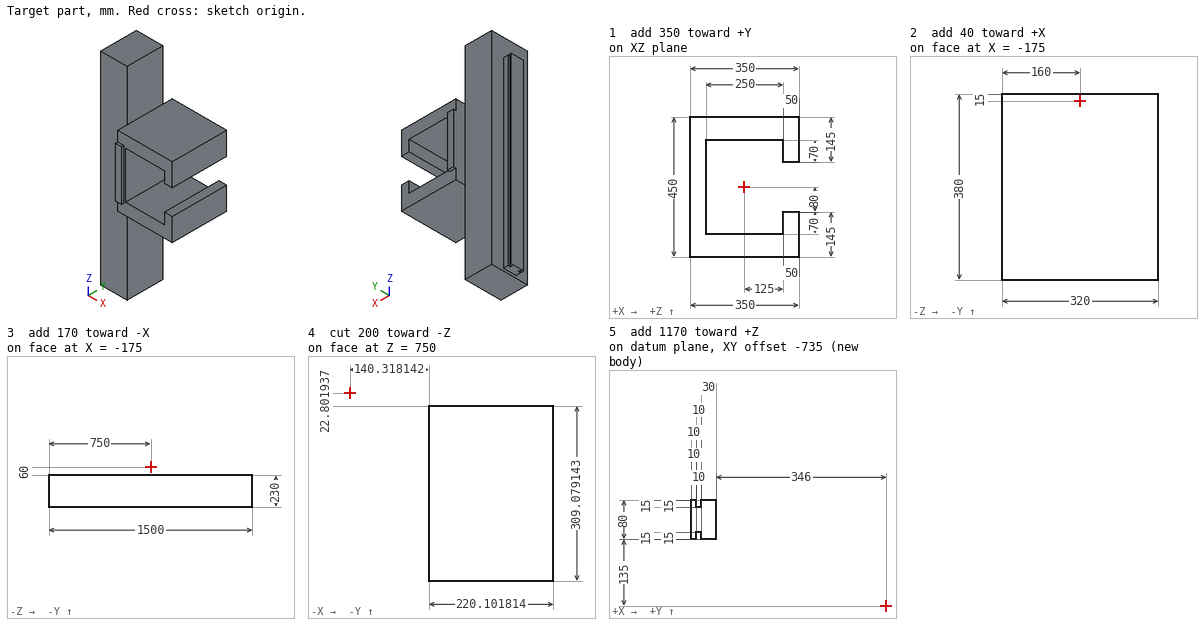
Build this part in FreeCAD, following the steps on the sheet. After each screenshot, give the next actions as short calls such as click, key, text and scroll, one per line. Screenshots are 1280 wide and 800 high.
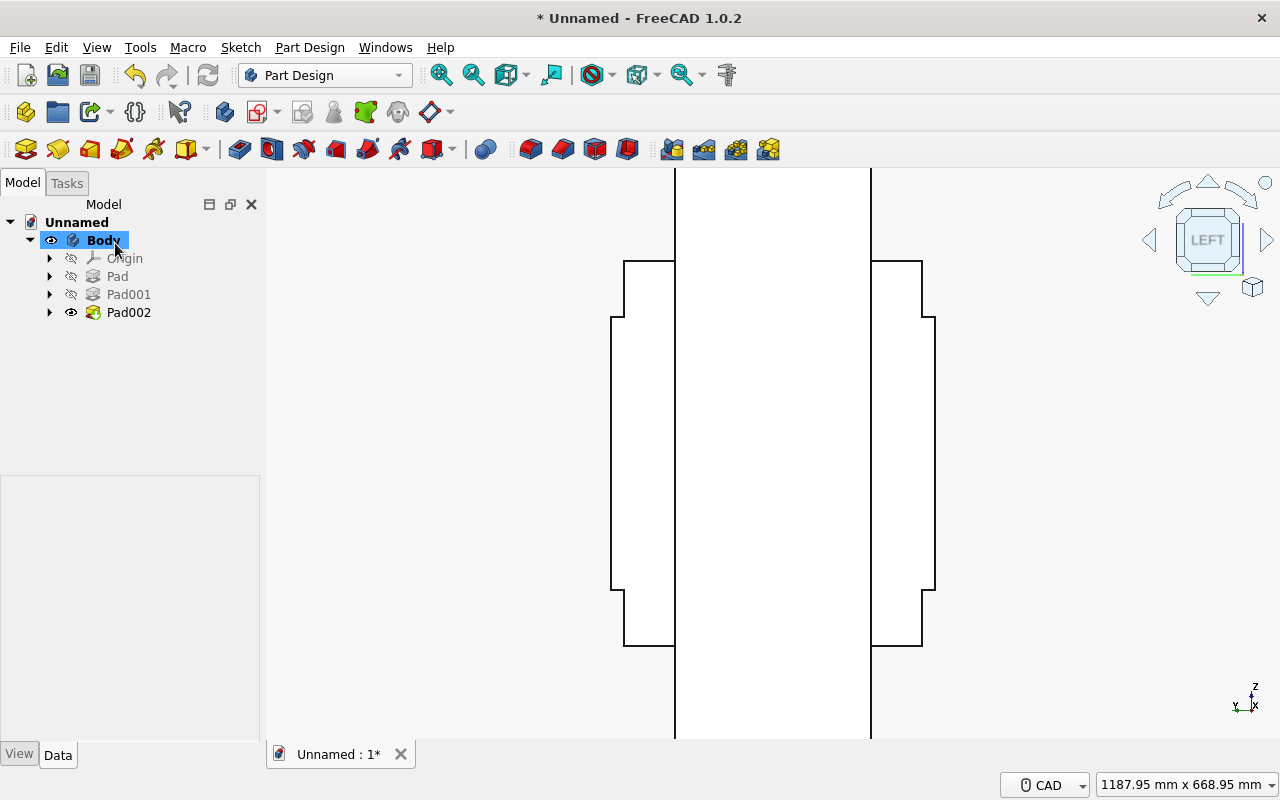
key(v)
key(f)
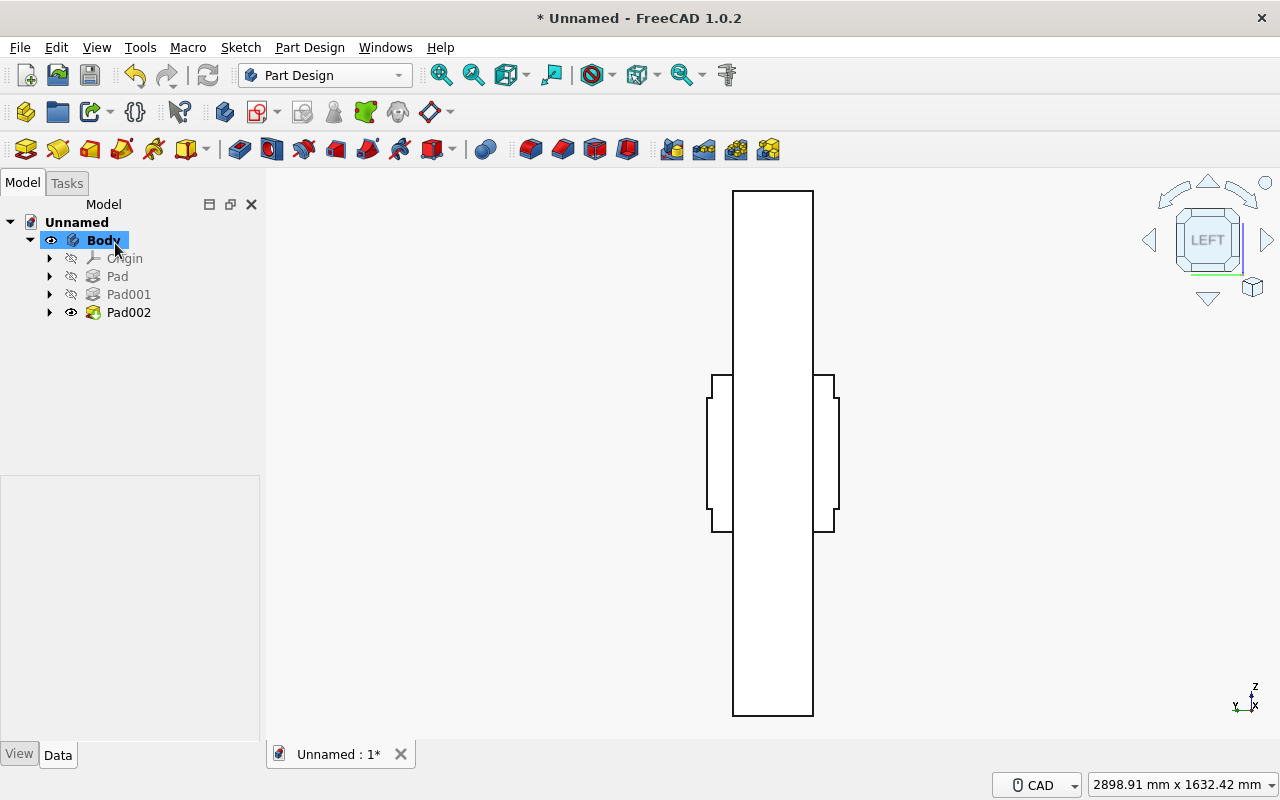
key(0)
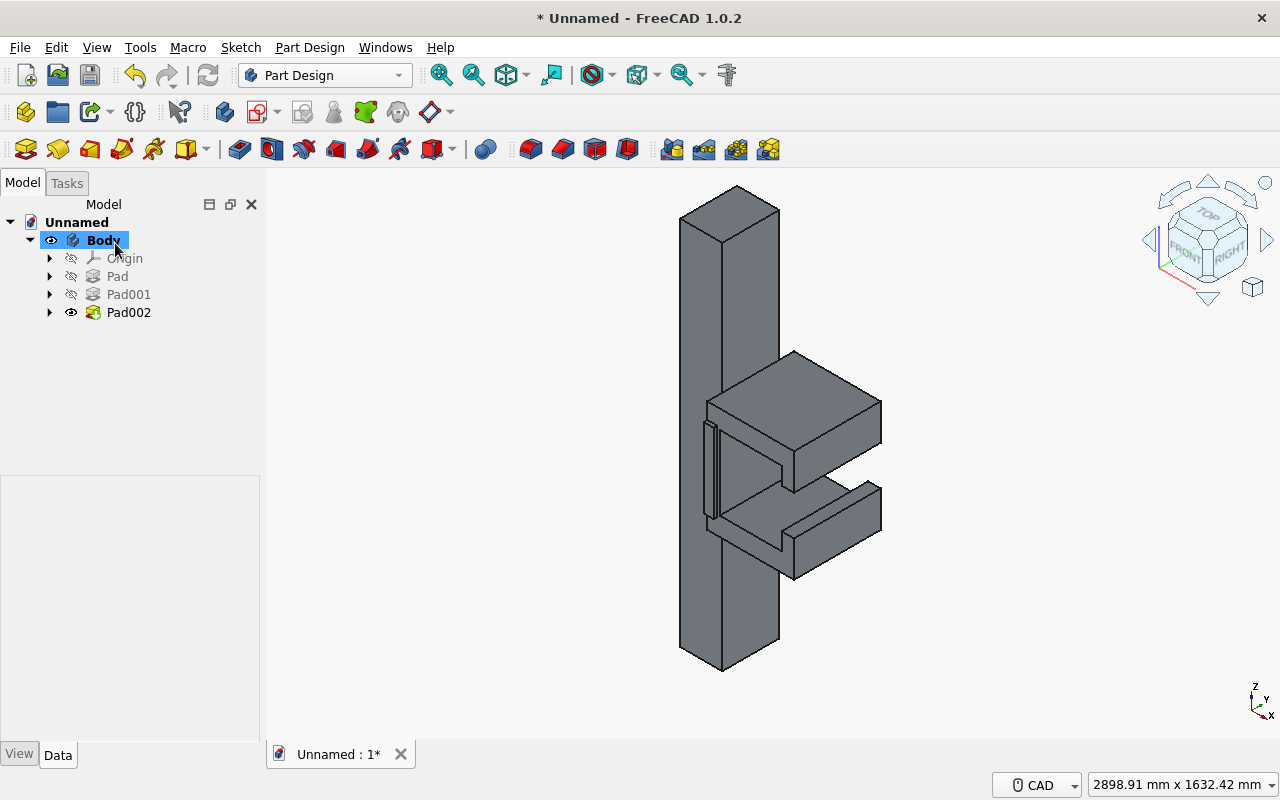
click(730, 213)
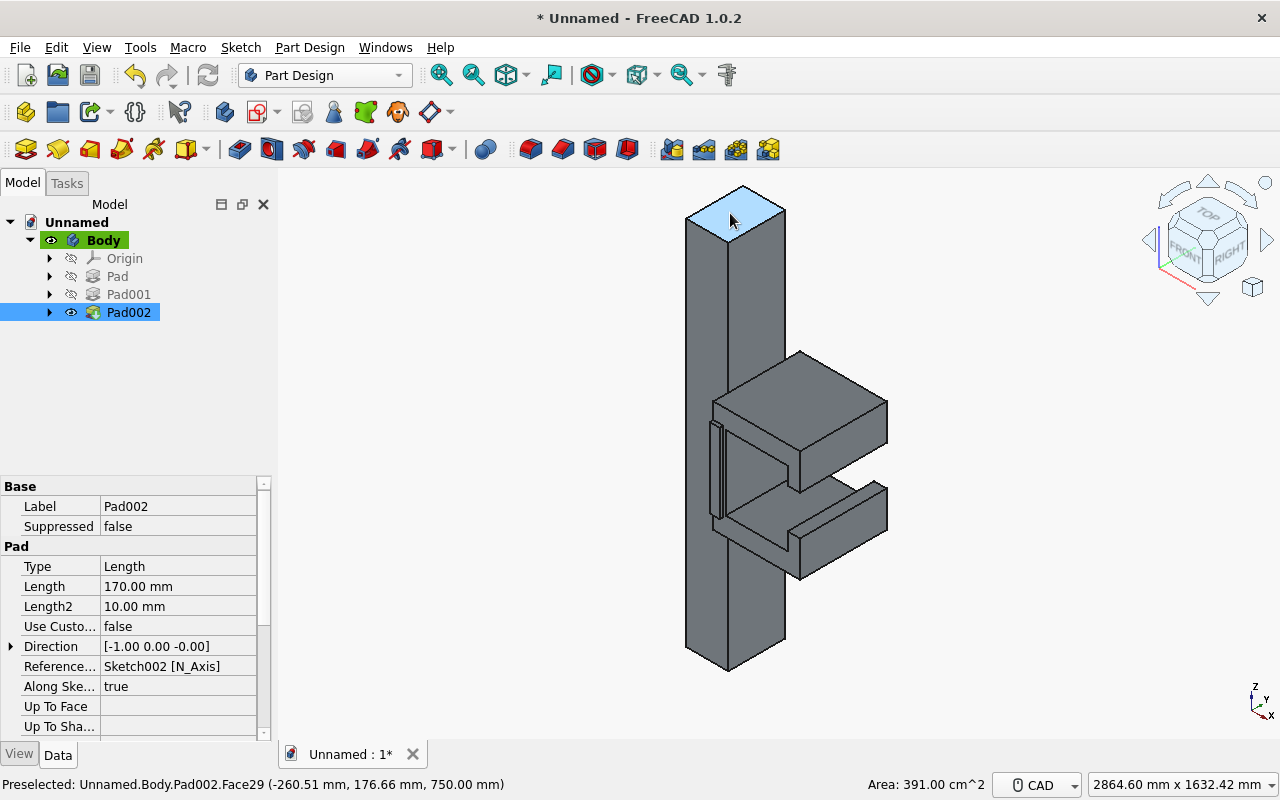
click(258, 112)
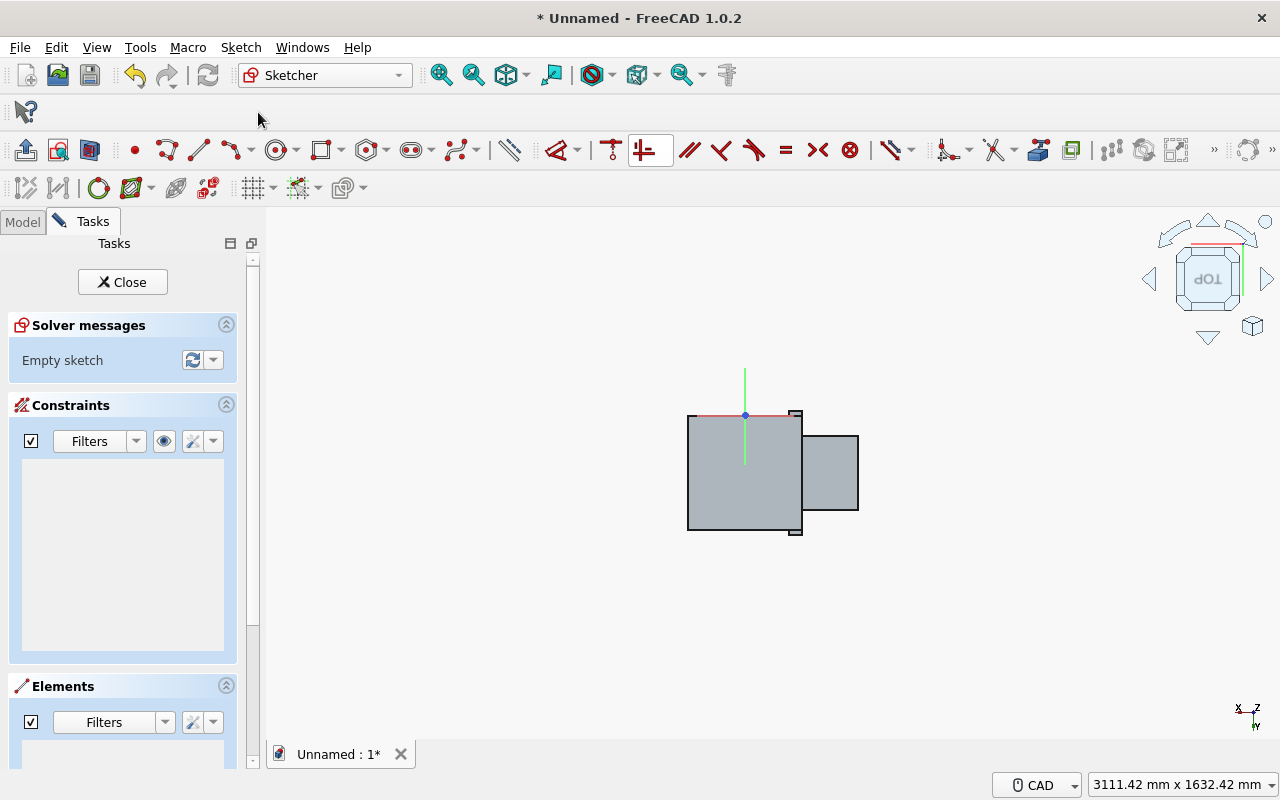
scroll(847, 469, up, 6)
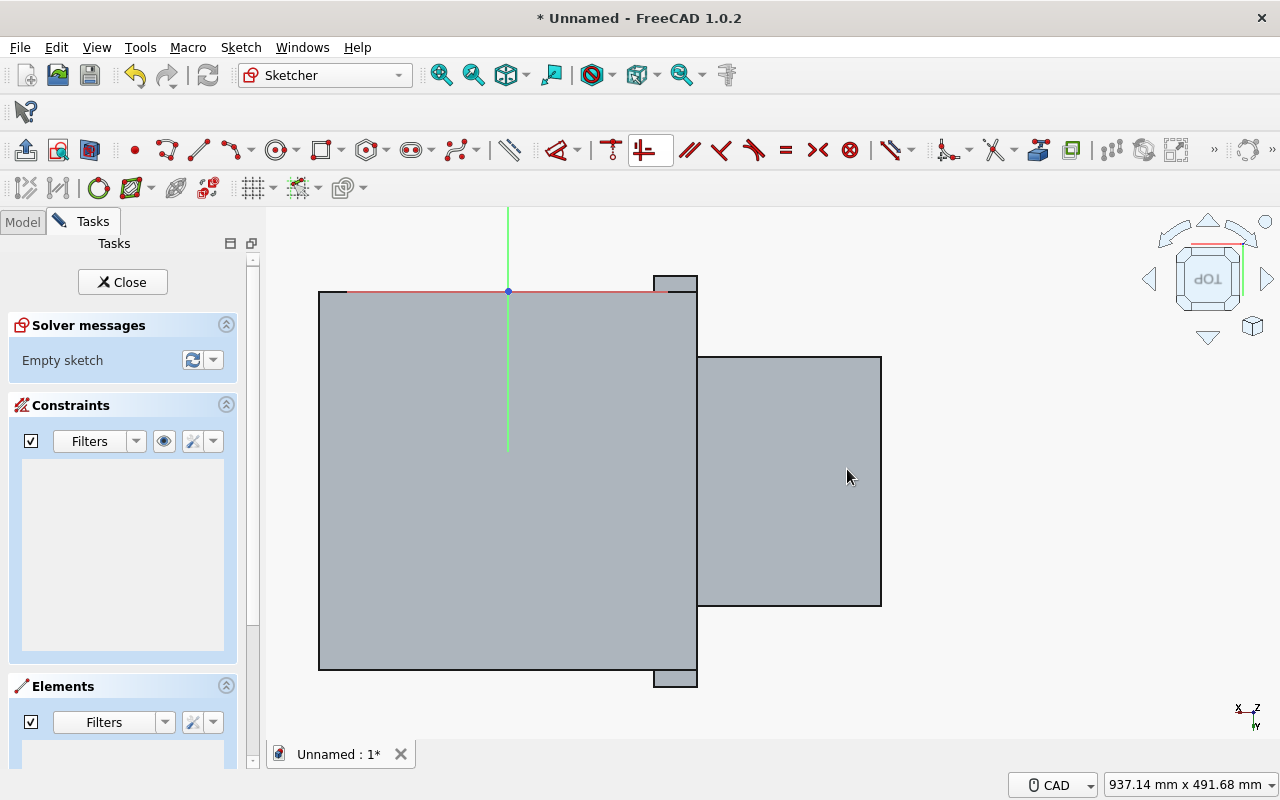
click(322, 150)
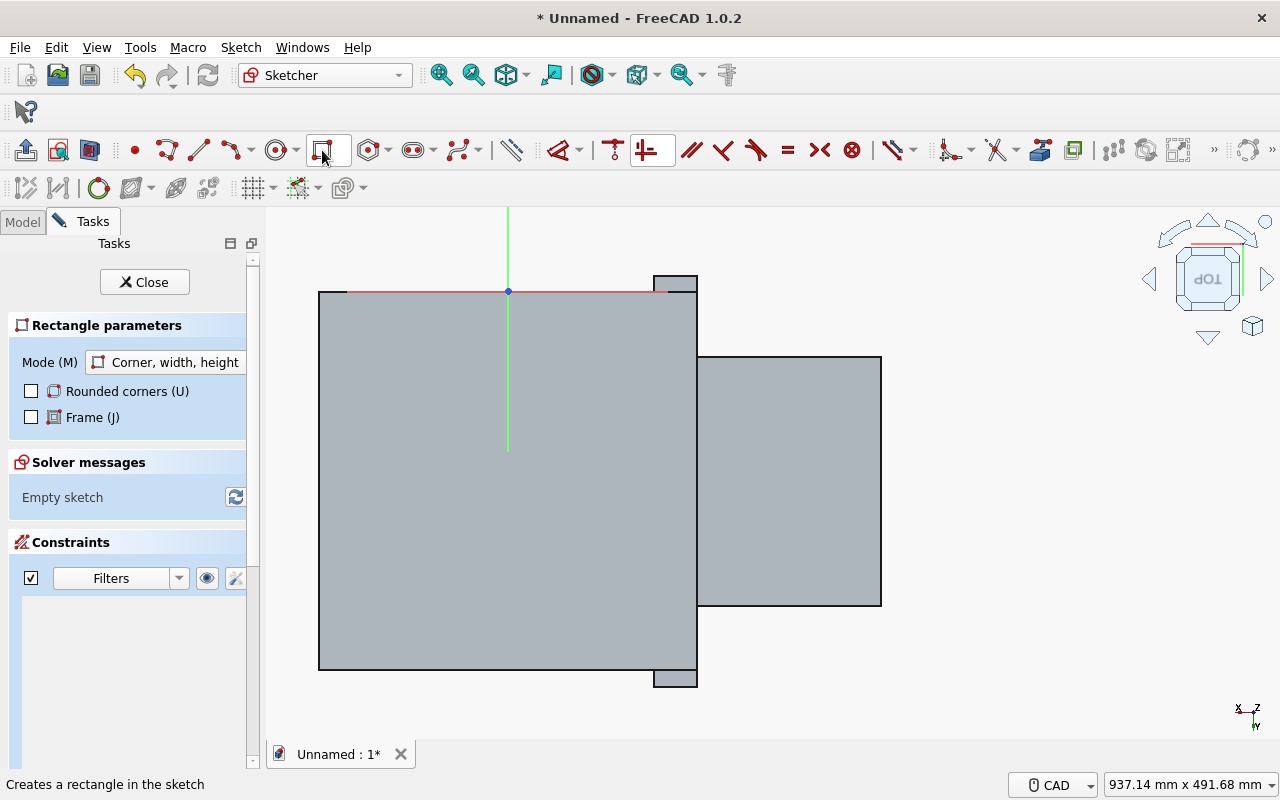
click(660, 316)
move(898, 651)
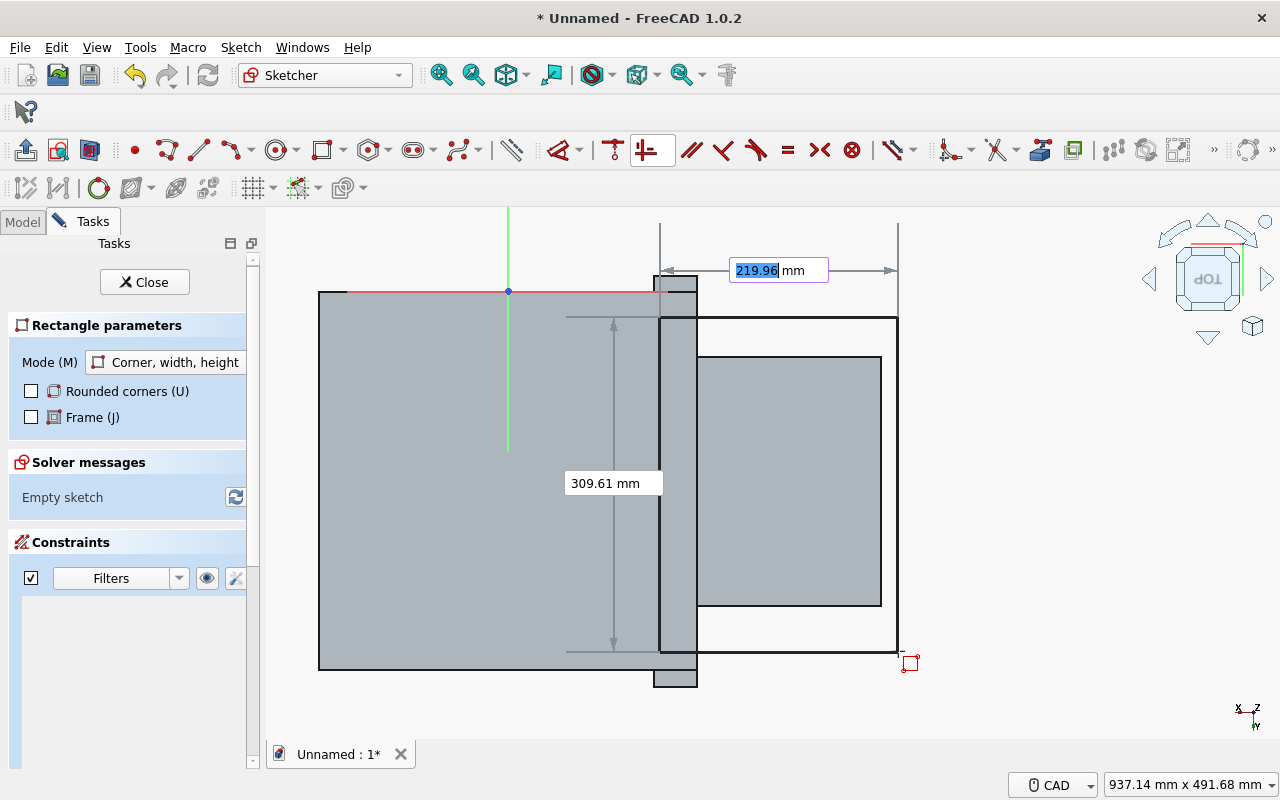
text(220.101814)
key(Tab)
text(309.079143)
key(Return)
key(Escape)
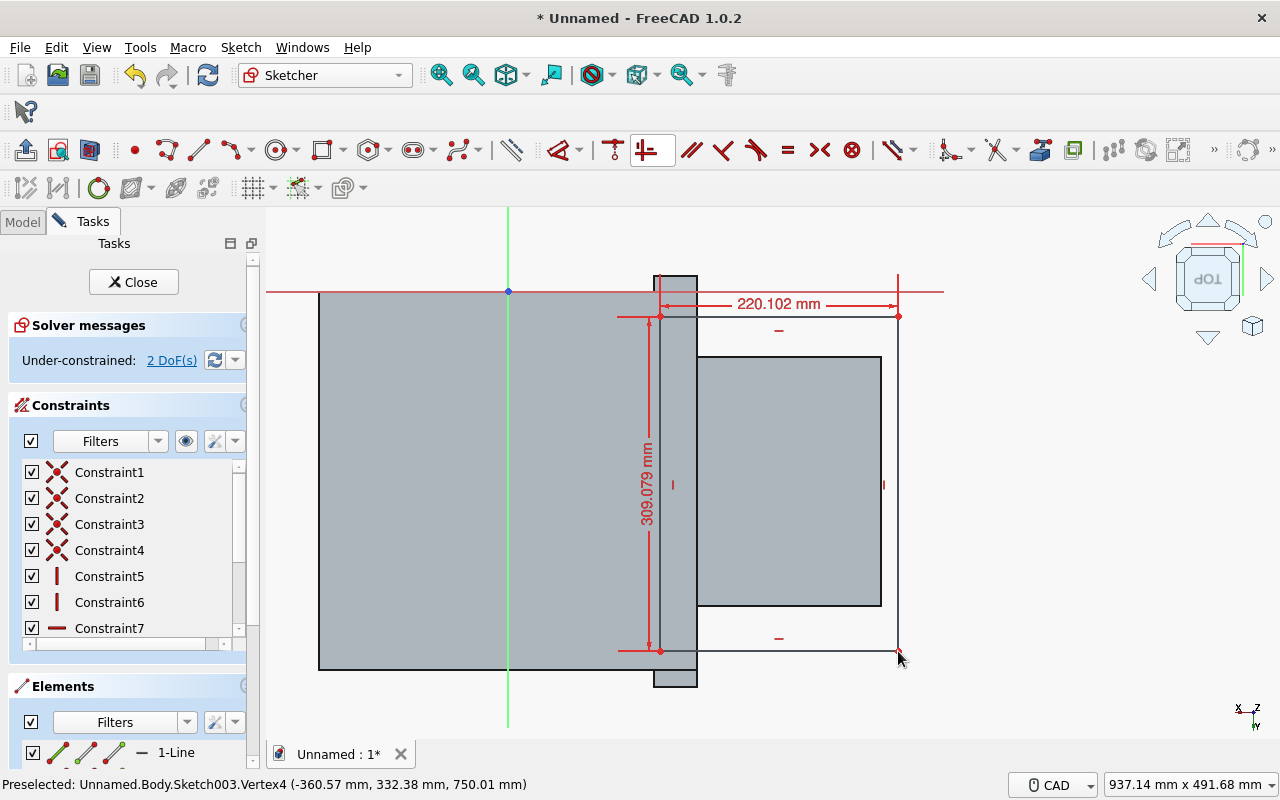
key(d)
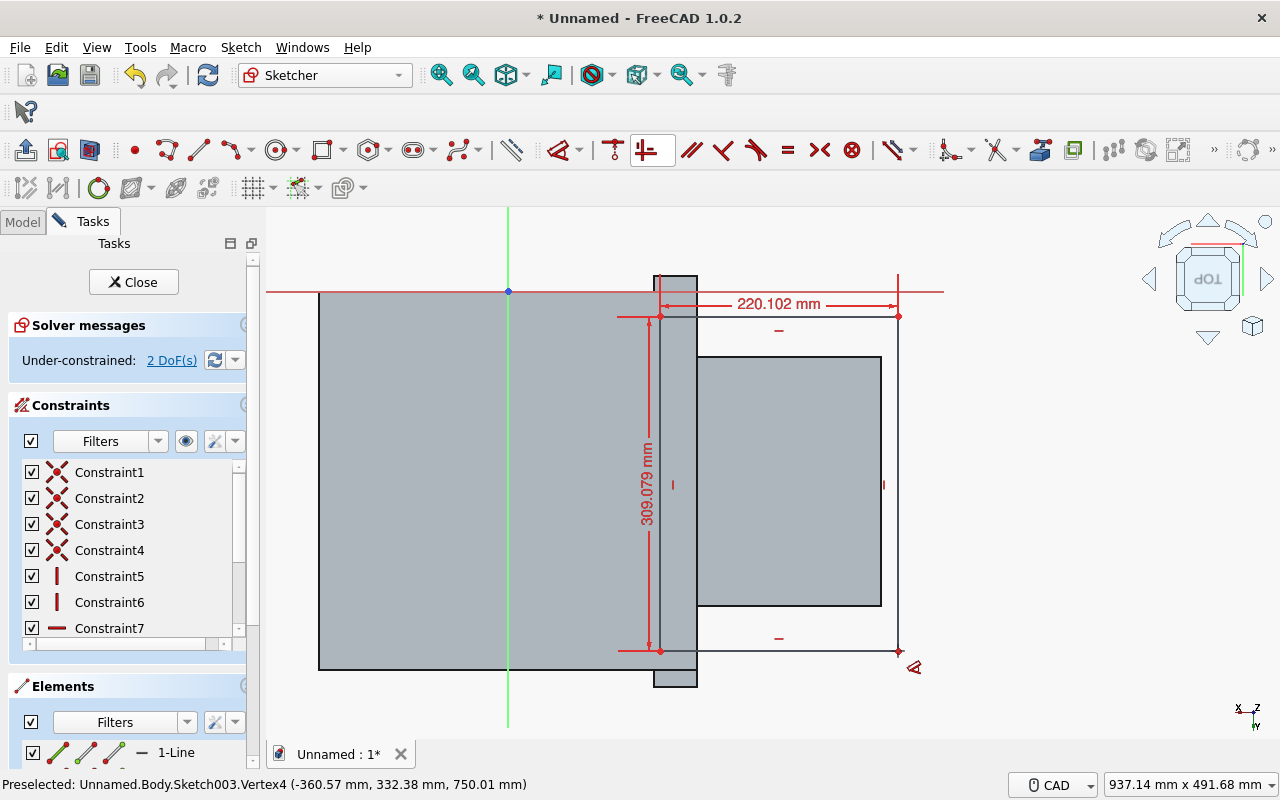
scroll(660, 317, up, 3)